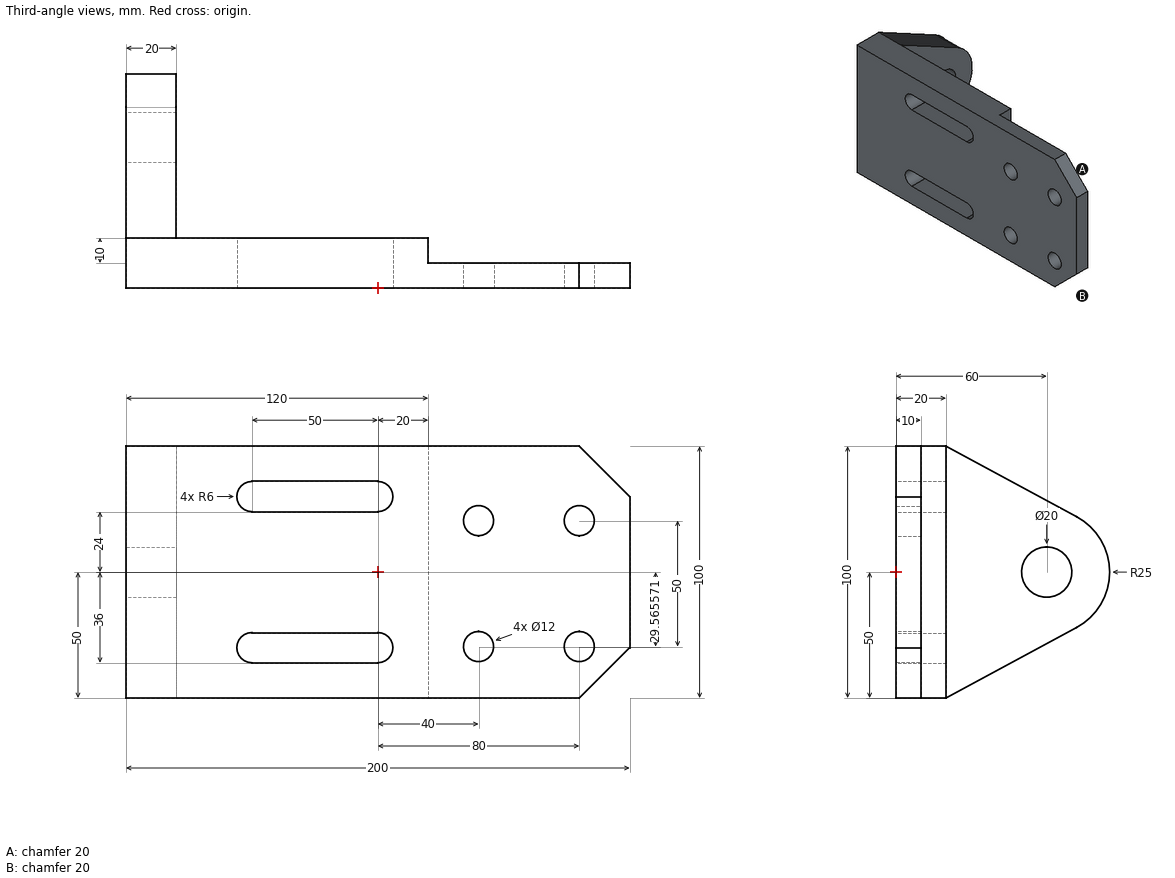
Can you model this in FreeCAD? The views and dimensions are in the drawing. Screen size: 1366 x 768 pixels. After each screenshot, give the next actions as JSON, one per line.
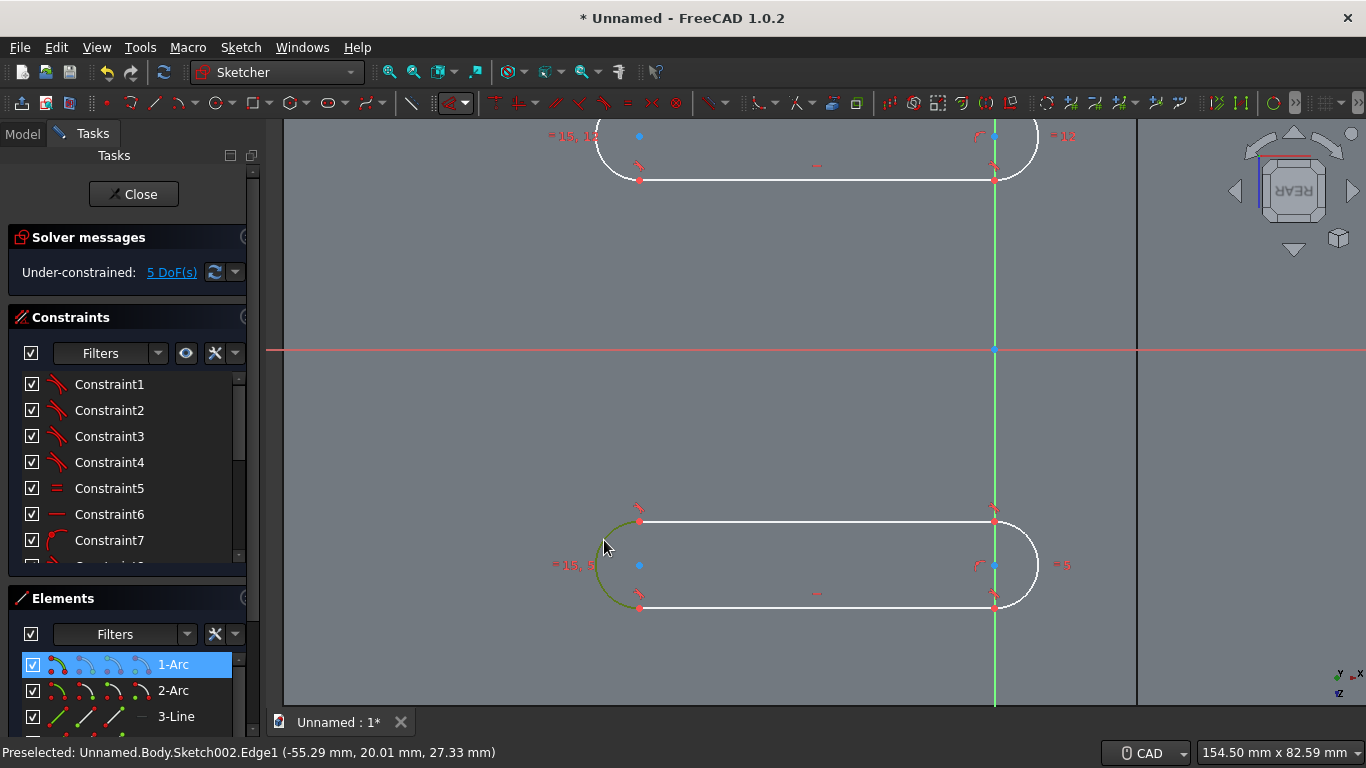
{"action": "key", "text": "k r"}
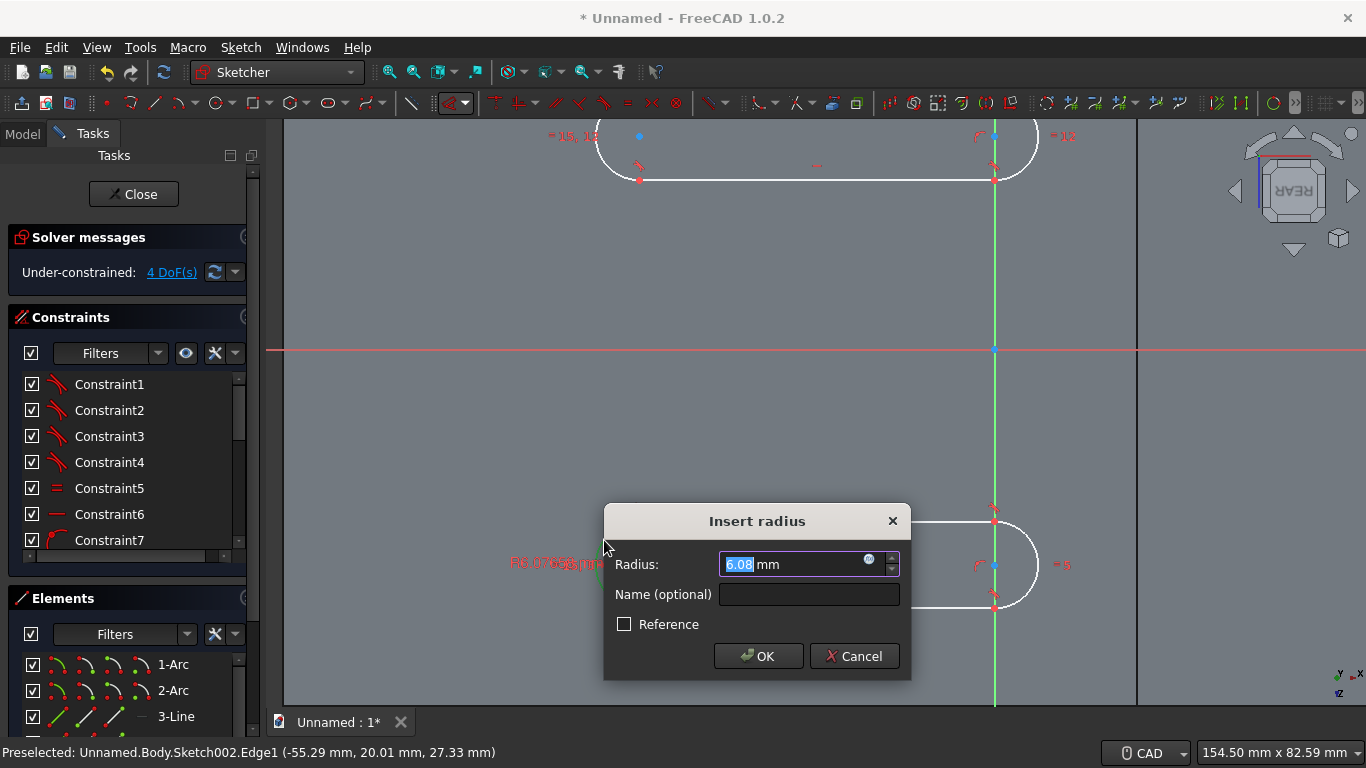
{"action": "type", "text": "6"}
{"action": "key", "text": "Return"}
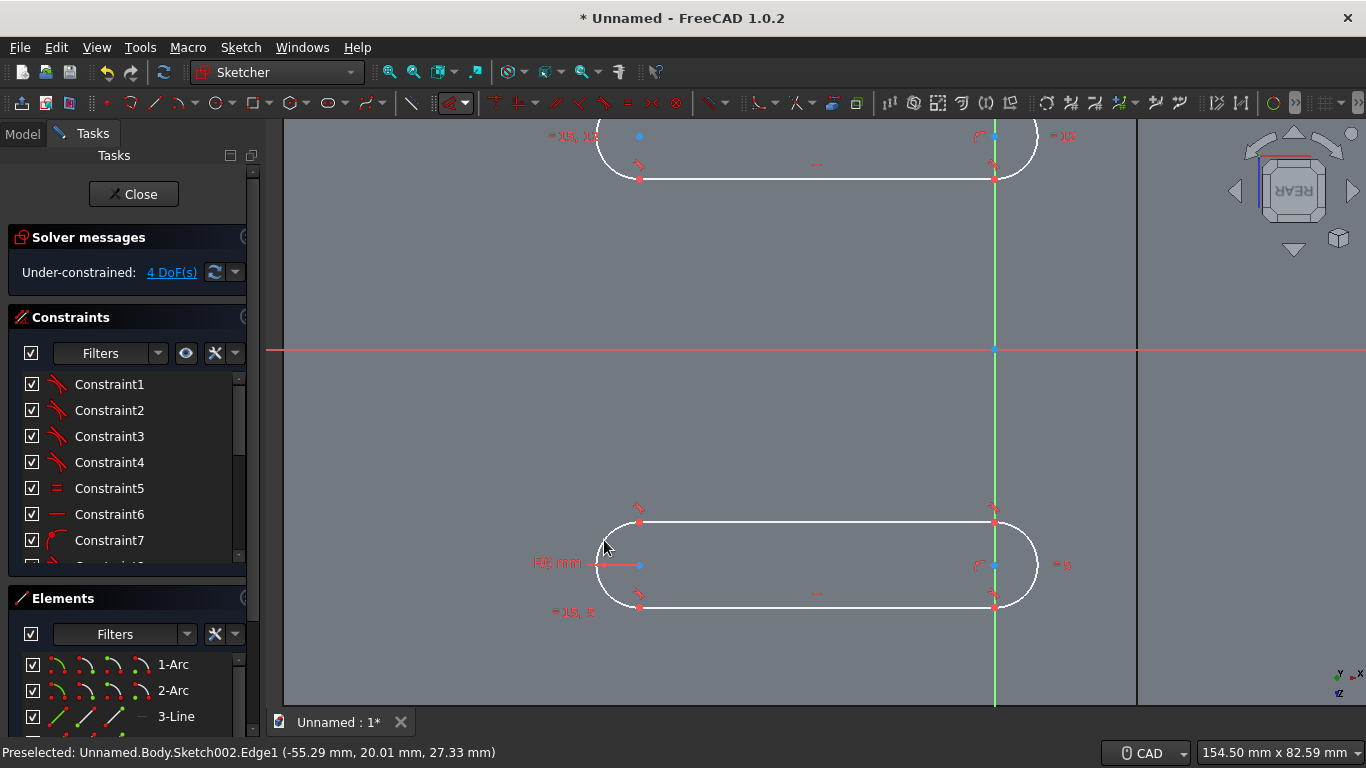
{"action": "left_click", "coordinate": [746, 522]}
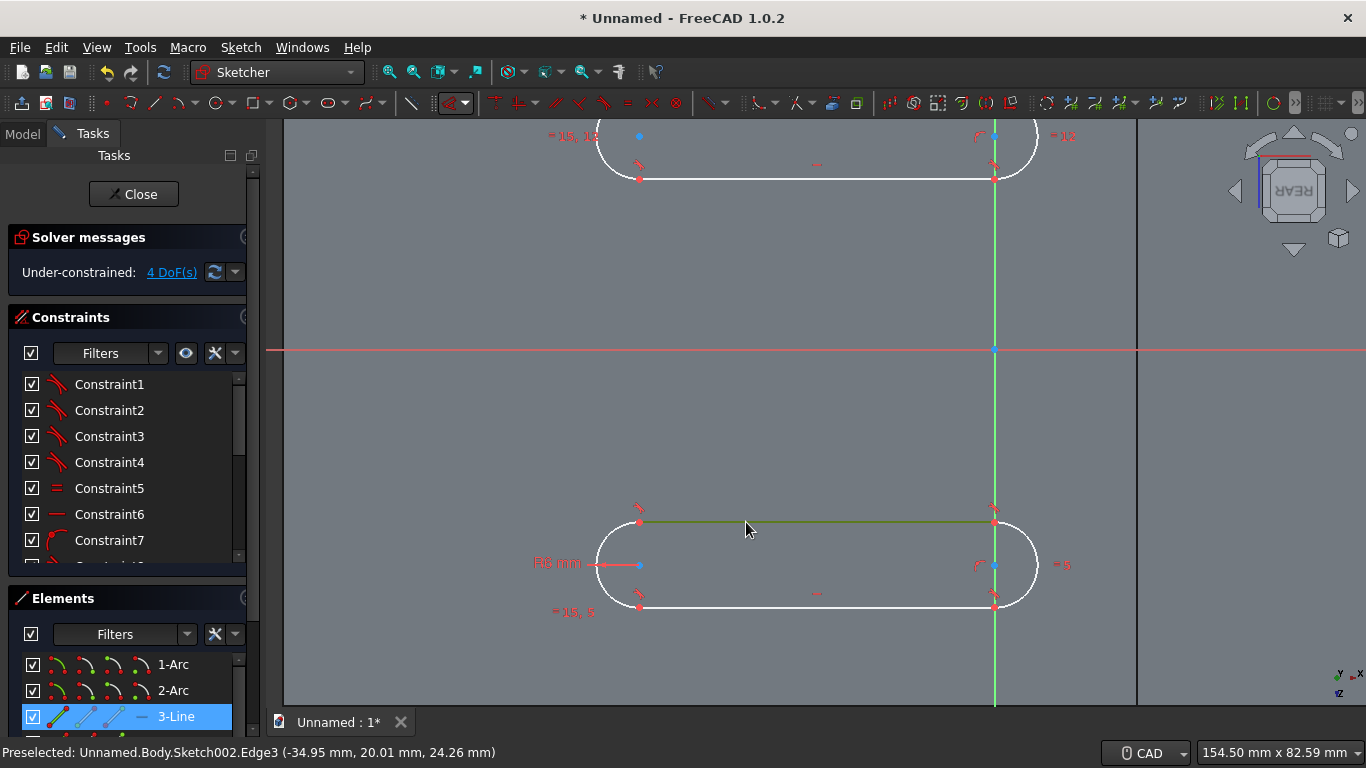
{"action": "left_click", "coordinate": [468, 104]}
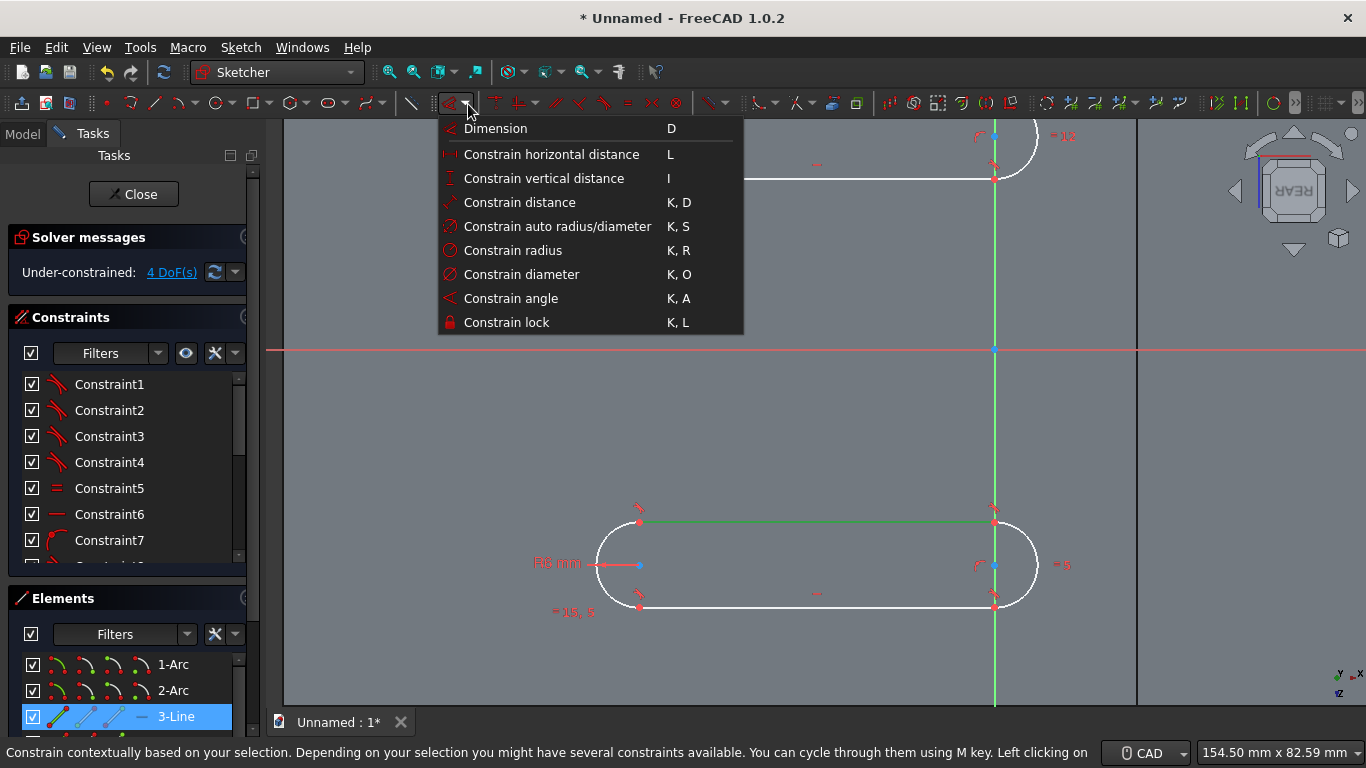
{"action": "left_click", "coordinate": [591, 154]}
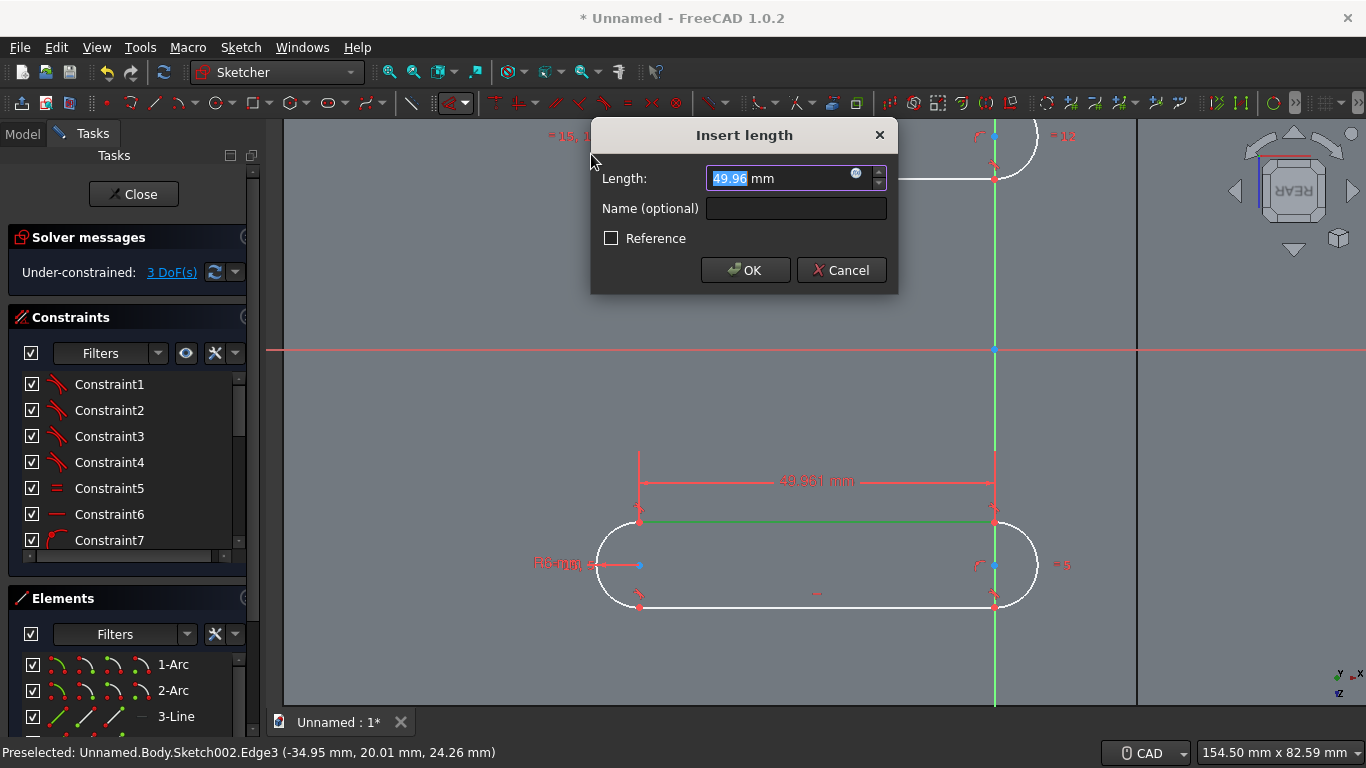
{"action": "type", "text": "50"}
{"action": "key", "text": "Return"}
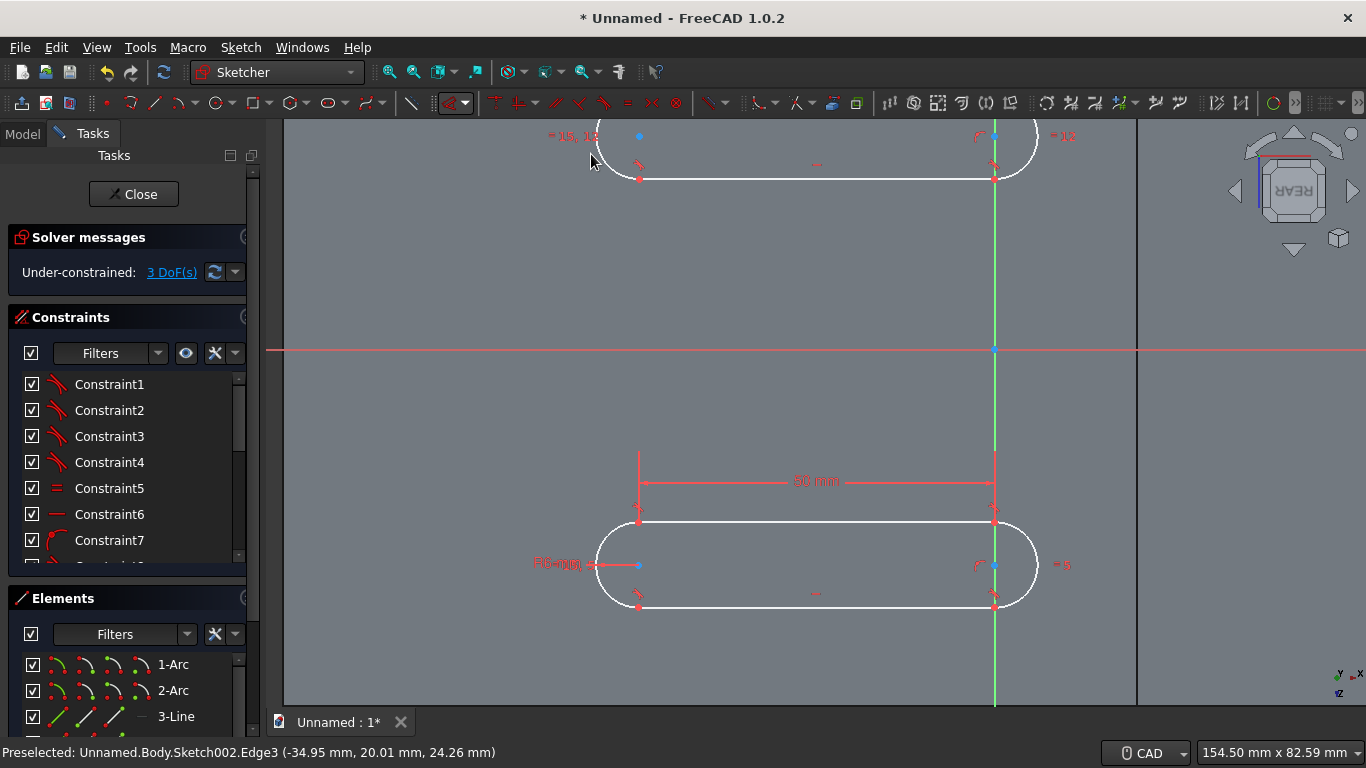
{"action": "scroll", "coordinate": [606, 542], "scroll_direction": "down", "scroll_amount": 2}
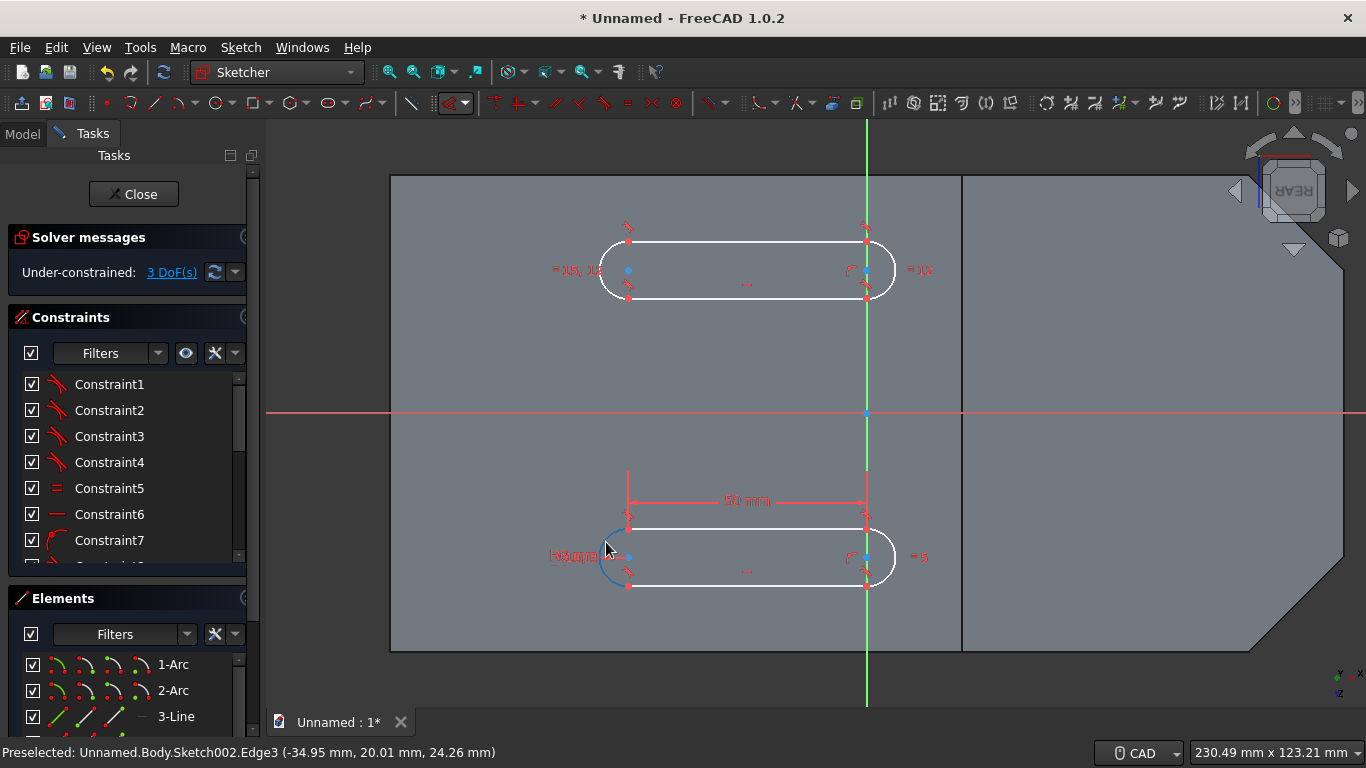
{"action": "left_click", "coordinate": [700, 242]}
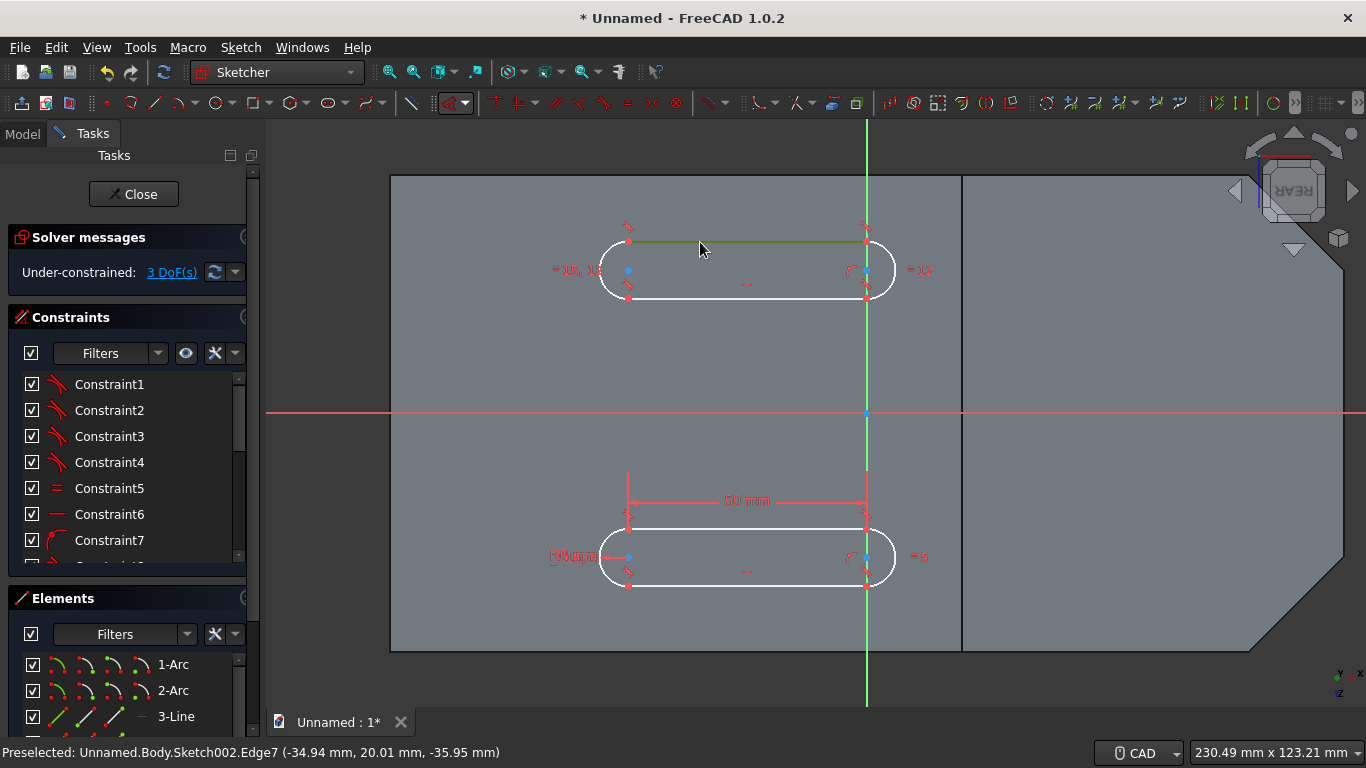
{"action": "left_click", "coordinate": [468, 104]}